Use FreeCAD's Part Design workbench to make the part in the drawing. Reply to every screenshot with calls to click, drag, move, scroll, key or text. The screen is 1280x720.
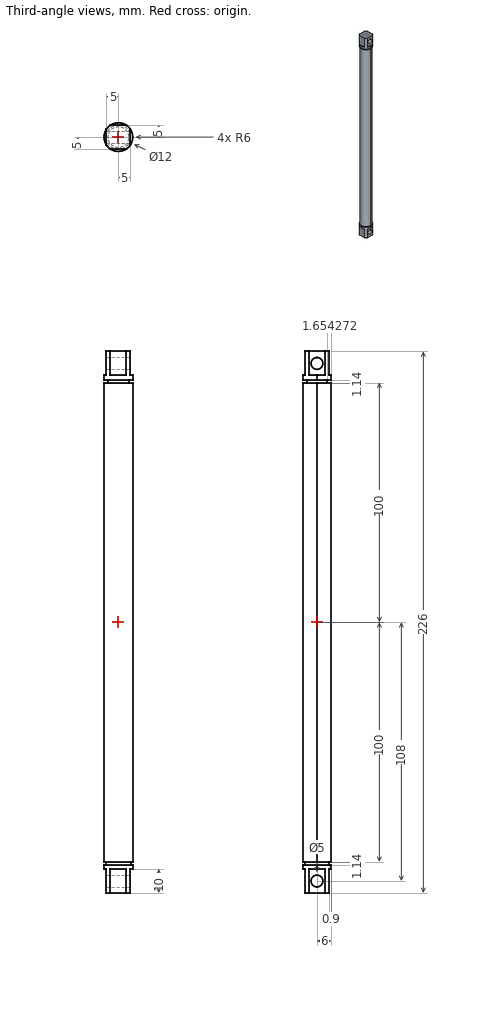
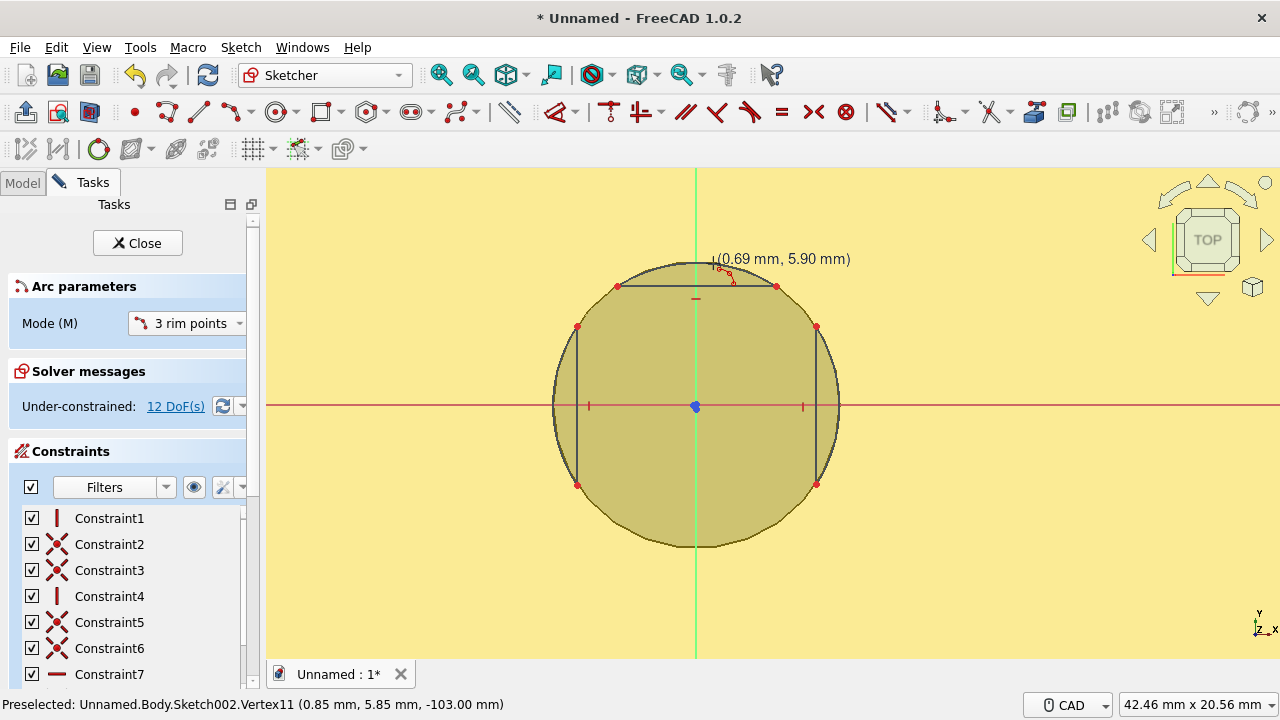
click(200, 112)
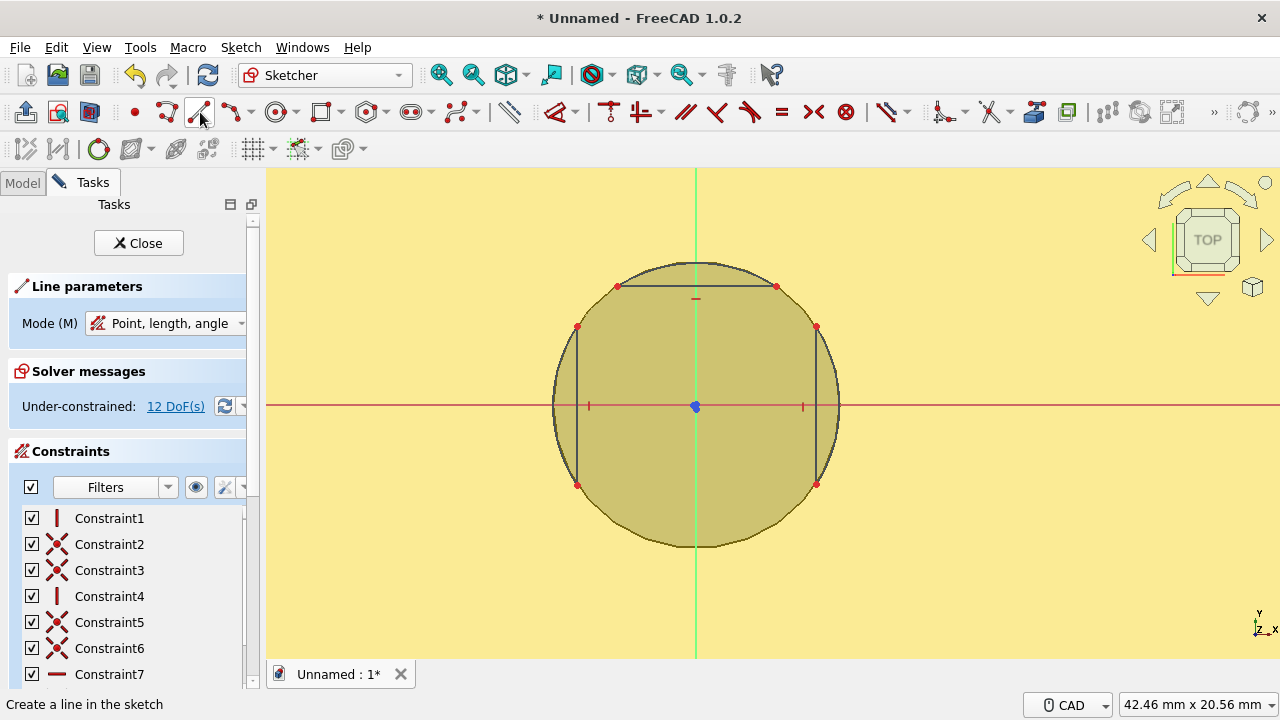
click(617, 524)
click(776, 524)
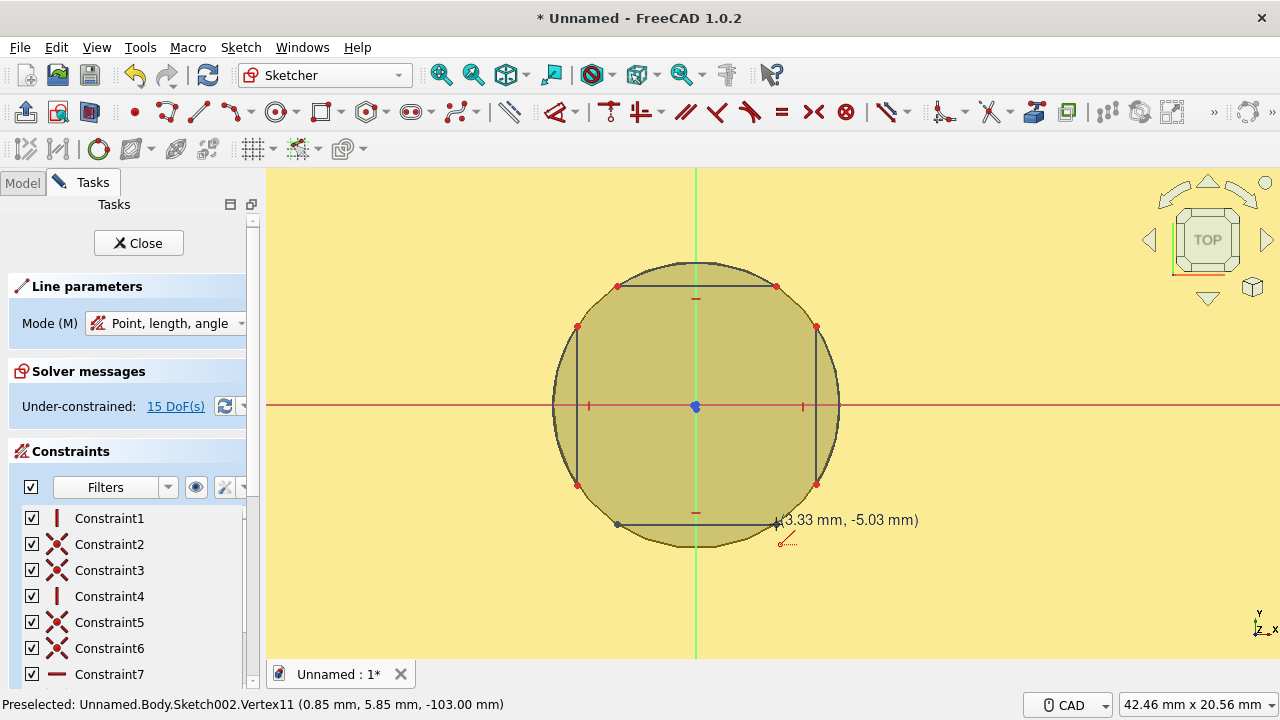
click(232, 112)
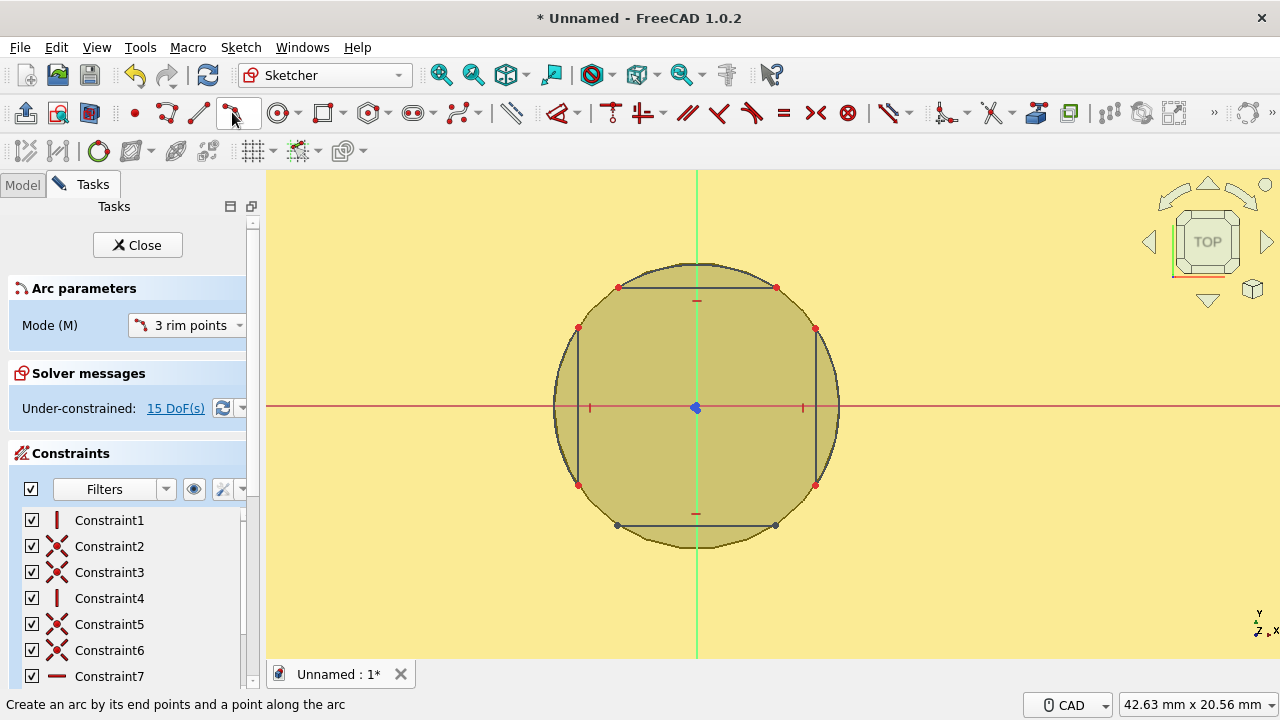
click(776, 526)
click(618, 526)
click(680, 548)
key(Escape)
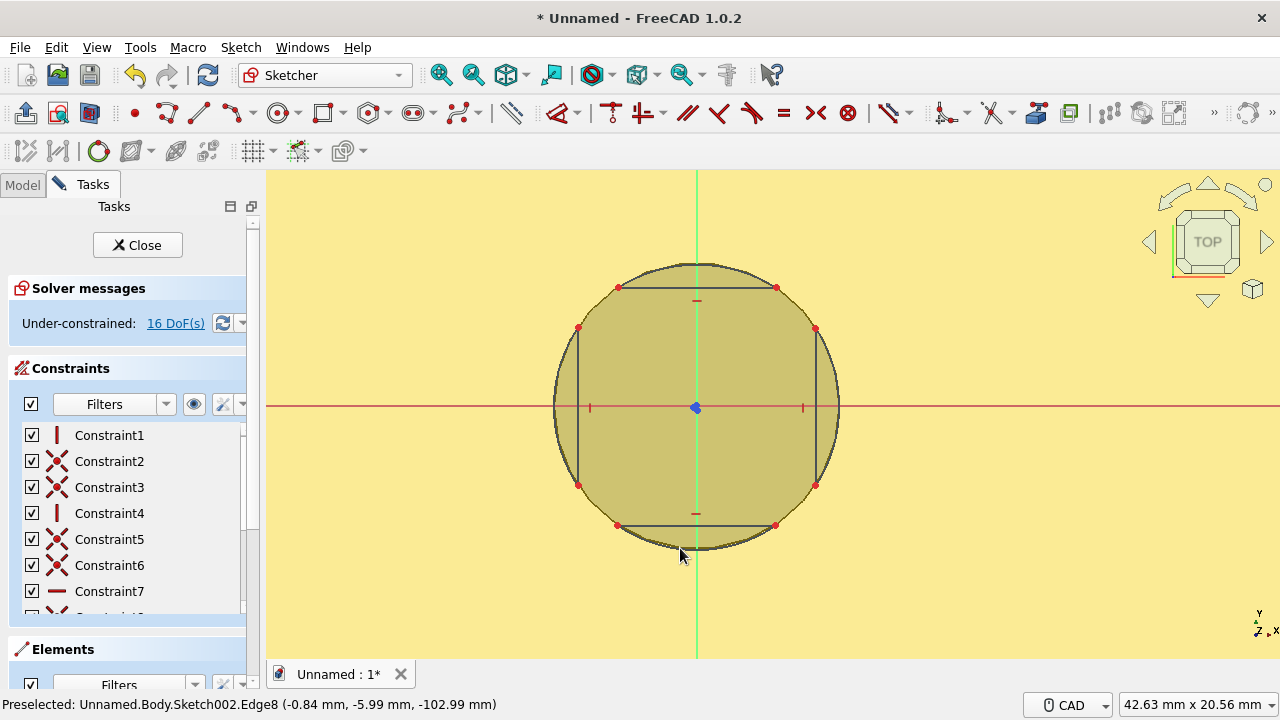
click(835, 440)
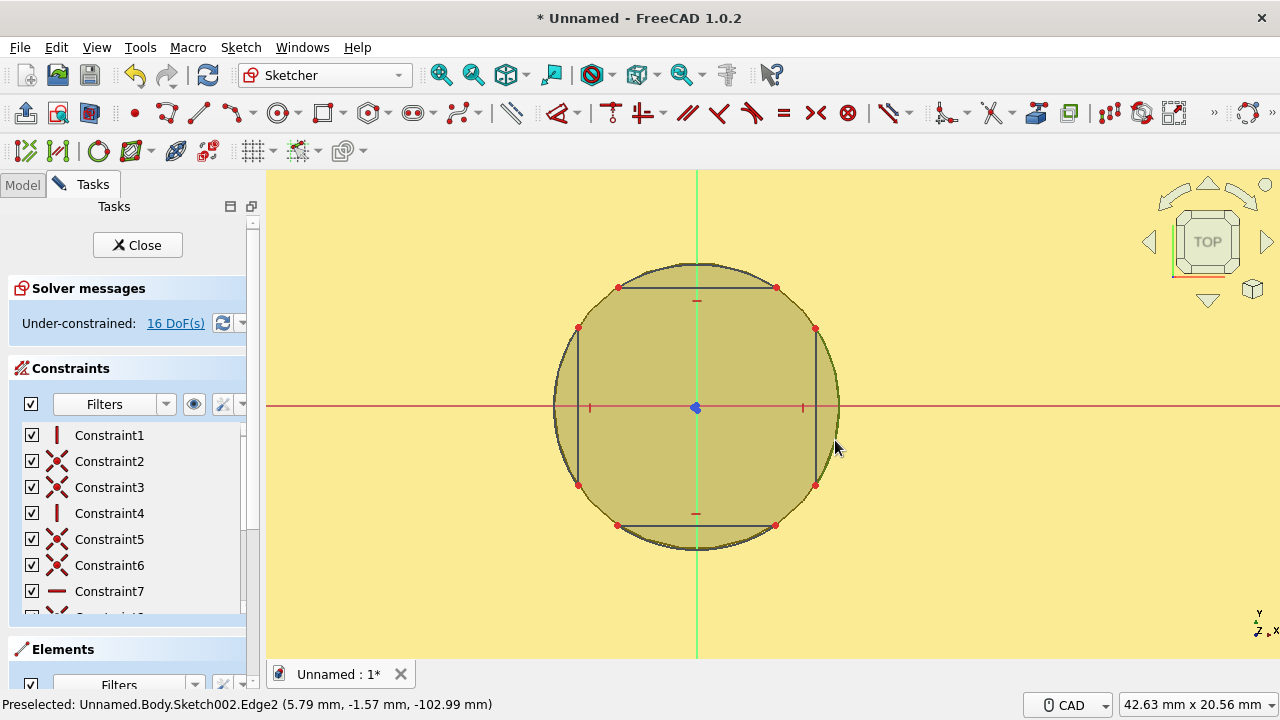
click(558, 374)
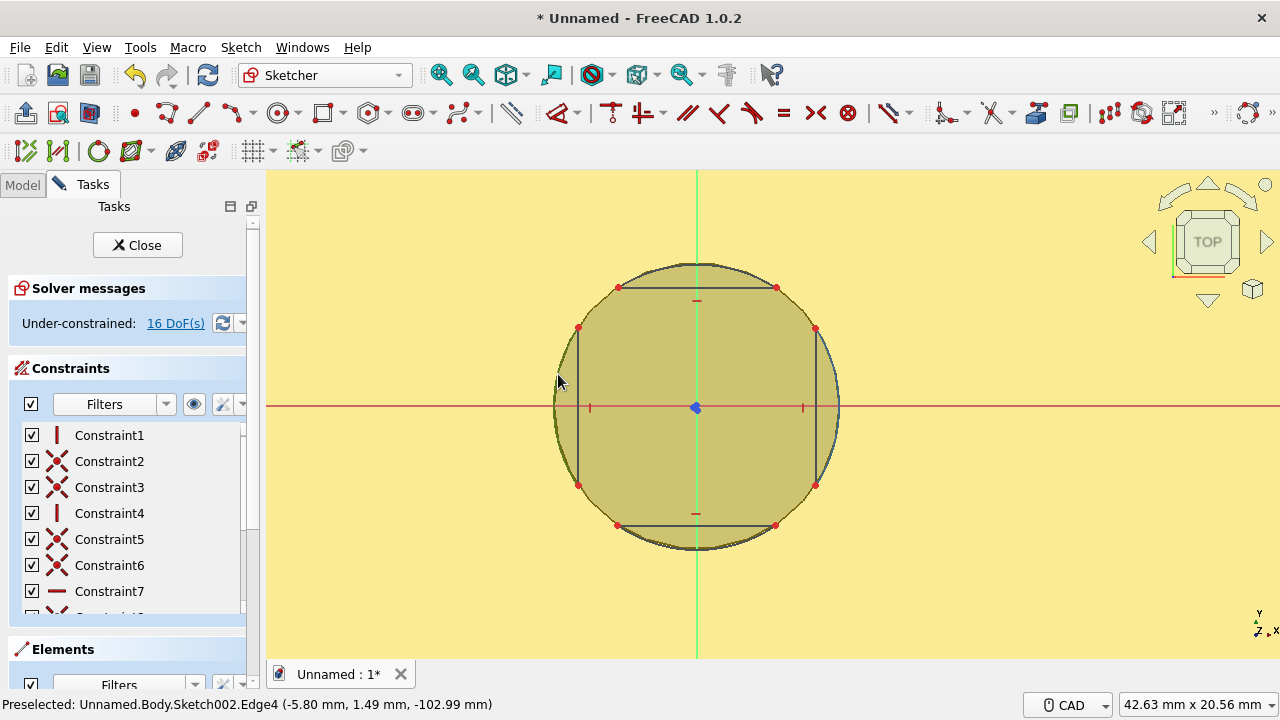
click(612, 114)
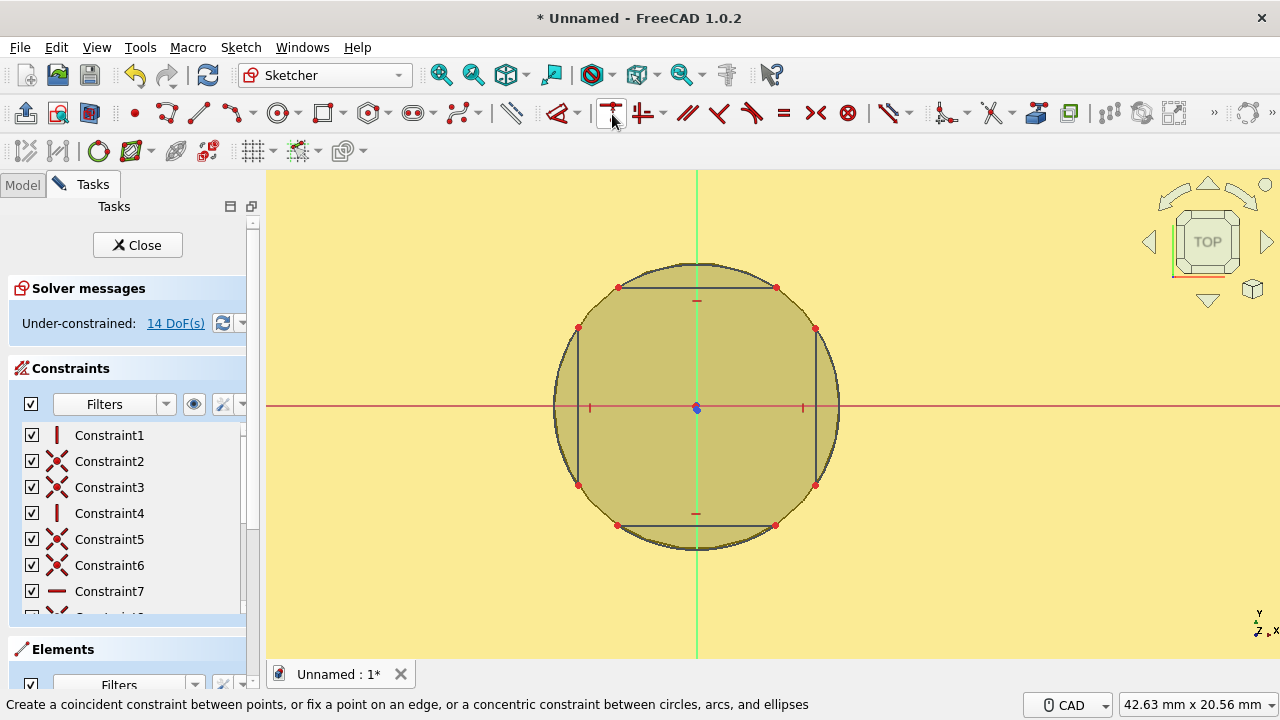
click(835, 440)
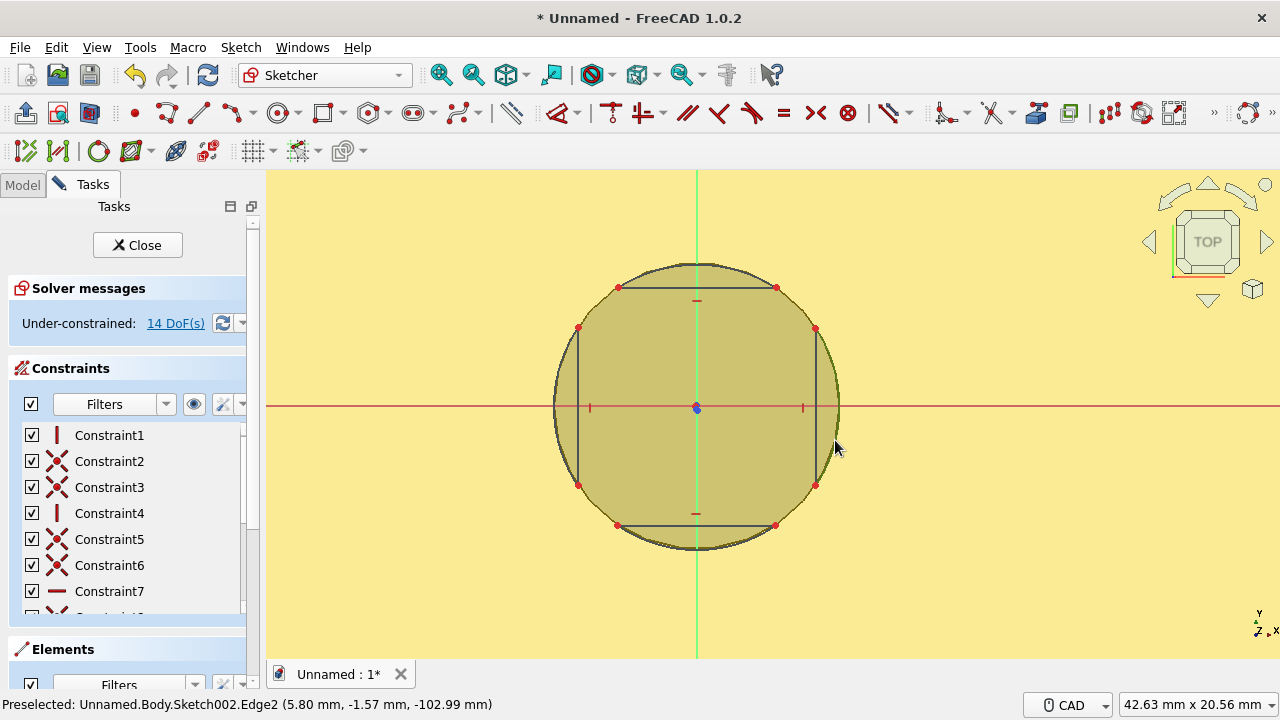
click(730, 269)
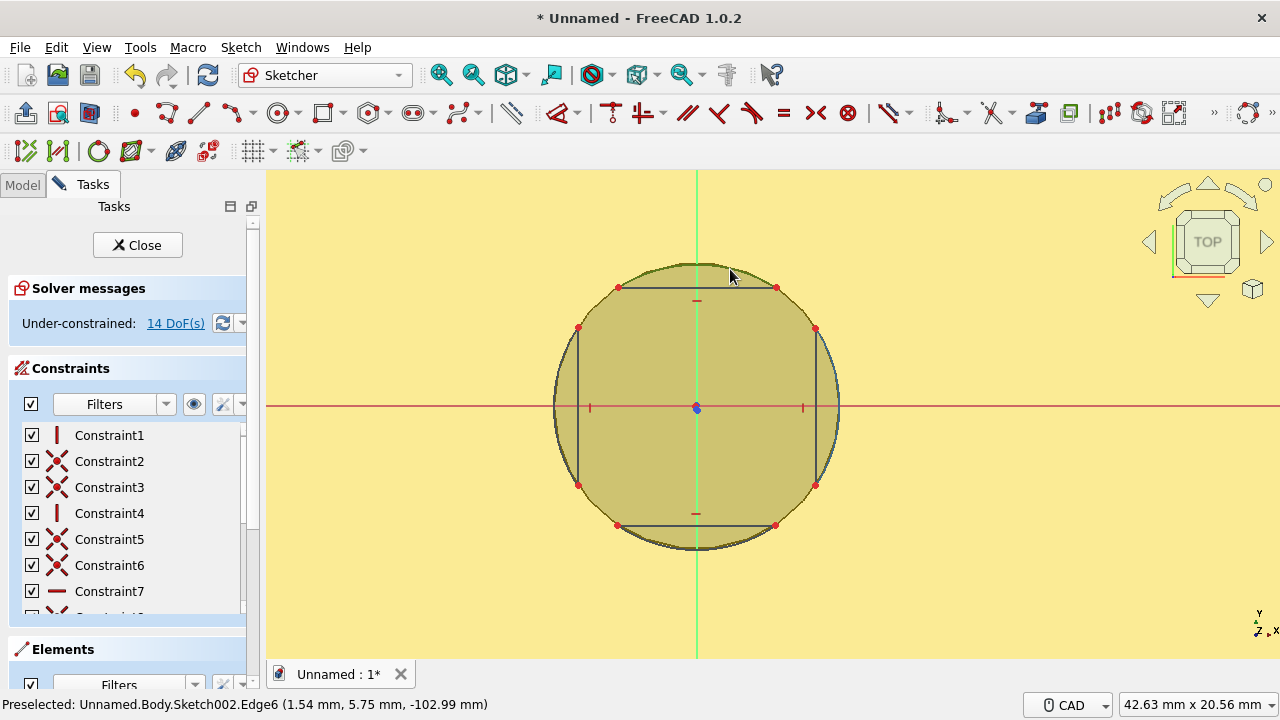
click(612, 114)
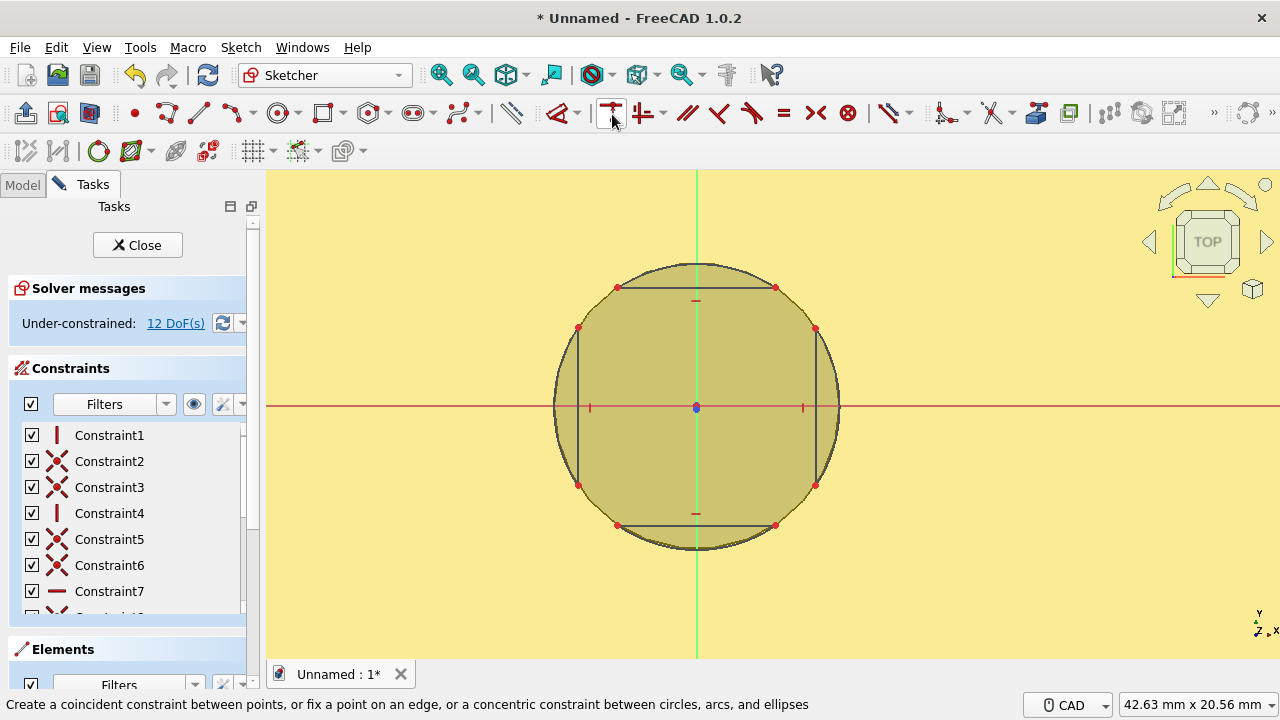
click(836, 440)